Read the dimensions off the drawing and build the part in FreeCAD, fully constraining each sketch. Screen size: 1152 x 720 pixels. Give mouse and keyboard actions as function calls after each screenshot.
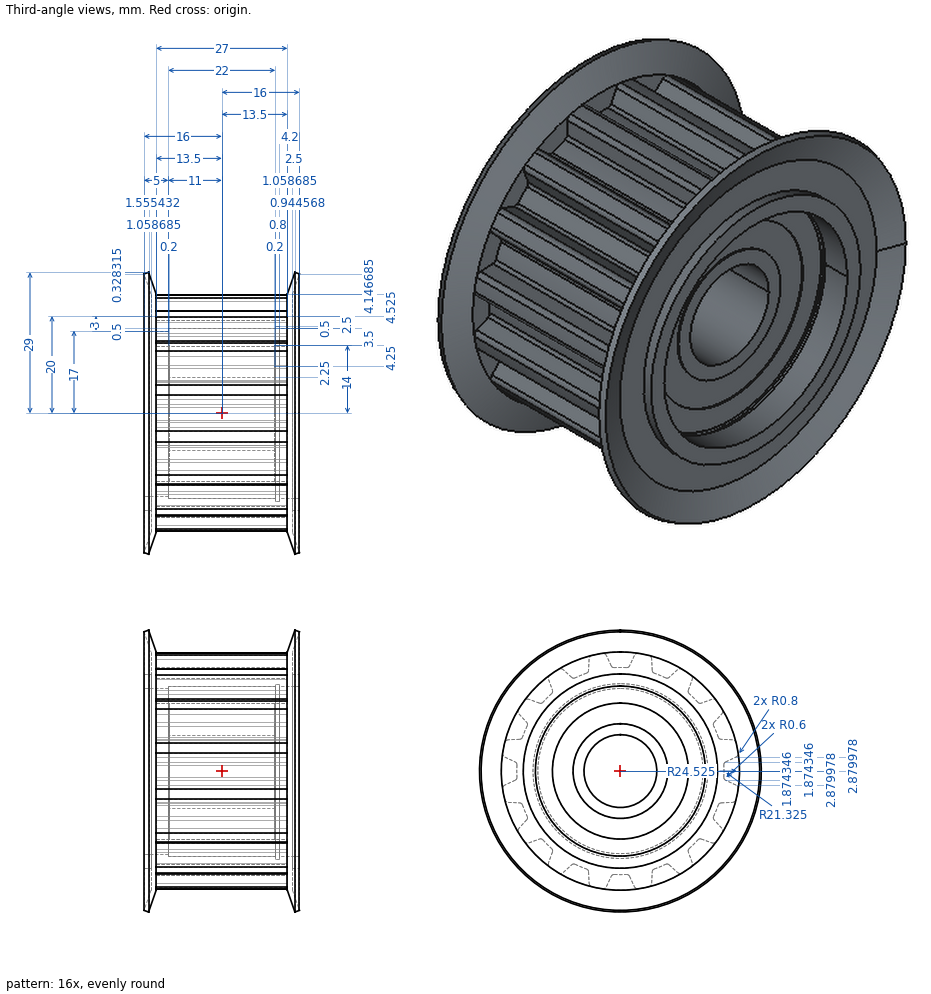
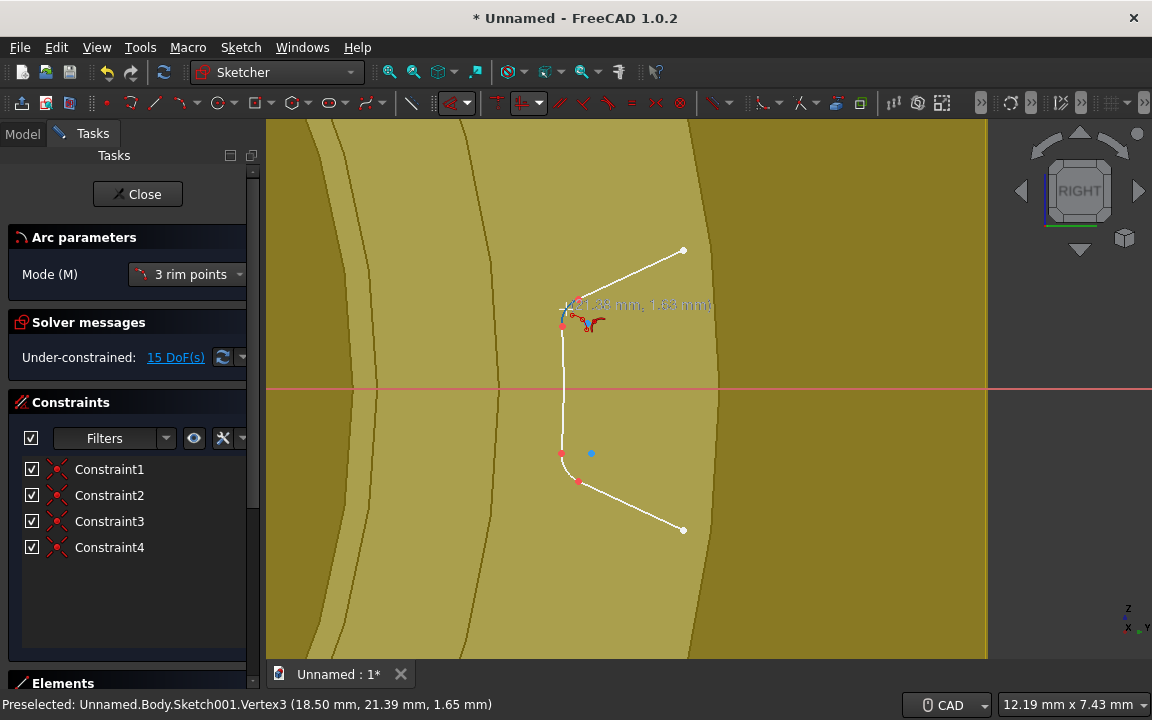
click(683, 250)
click(706, 208)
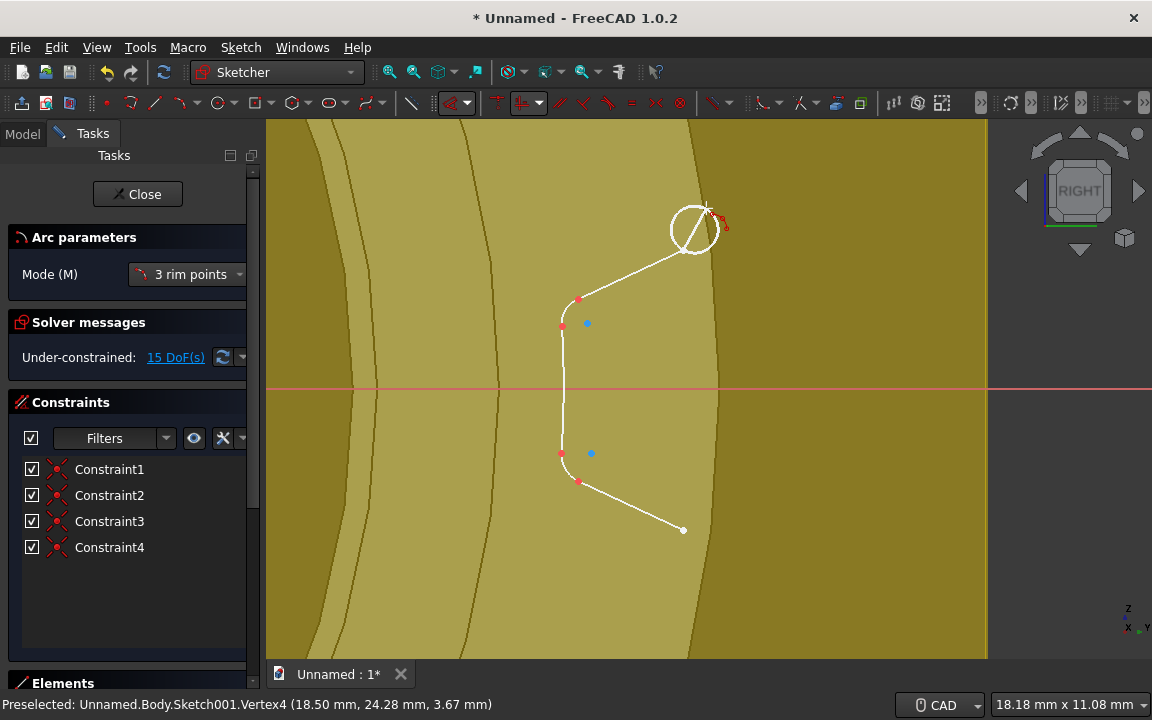
scroll(702, 232, up, 4)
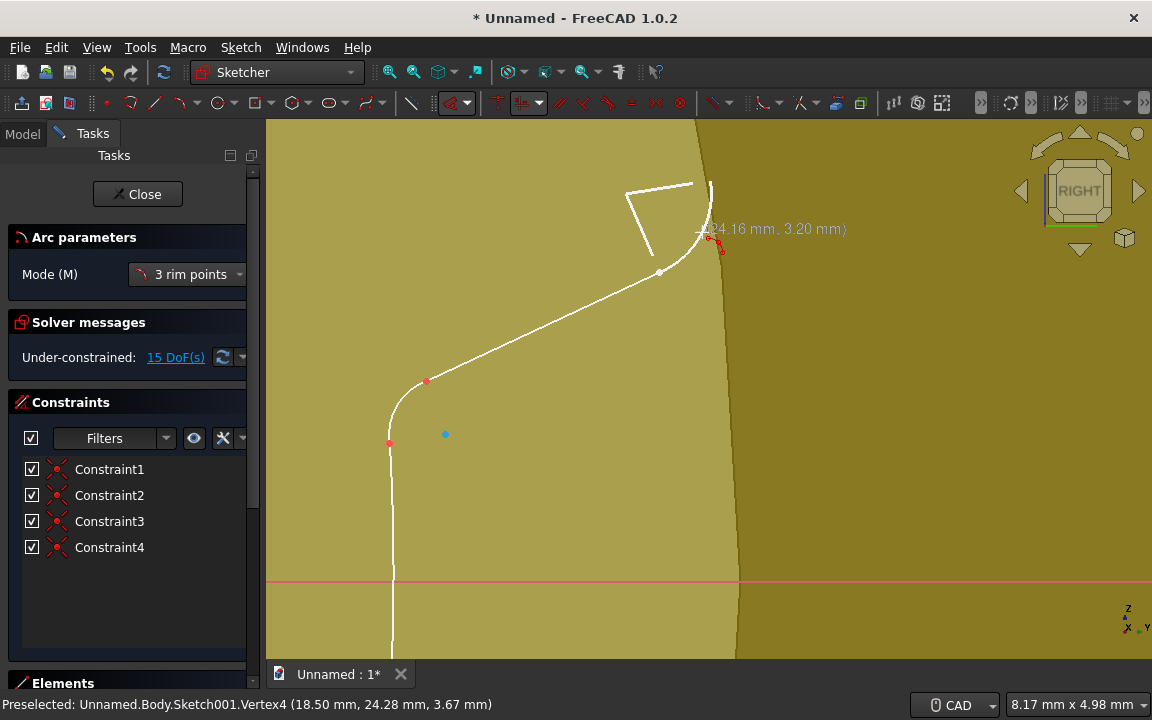
click(700, 231)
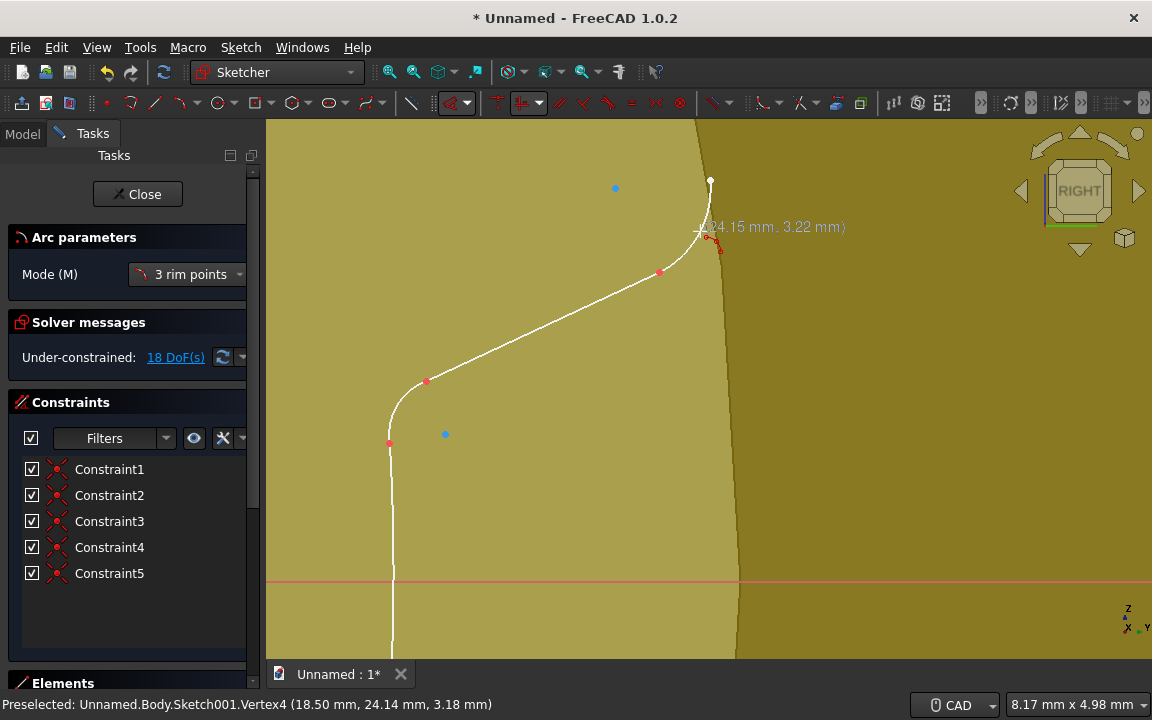
click(710, 181)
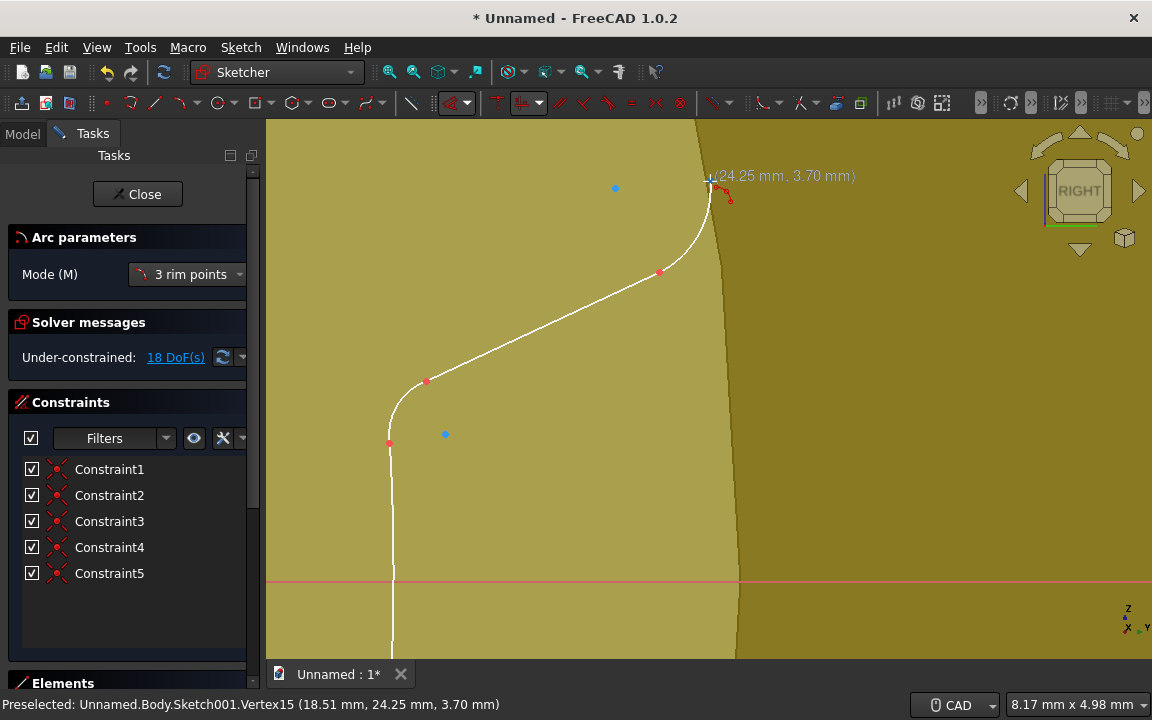
scroll(702, 232, down, 4)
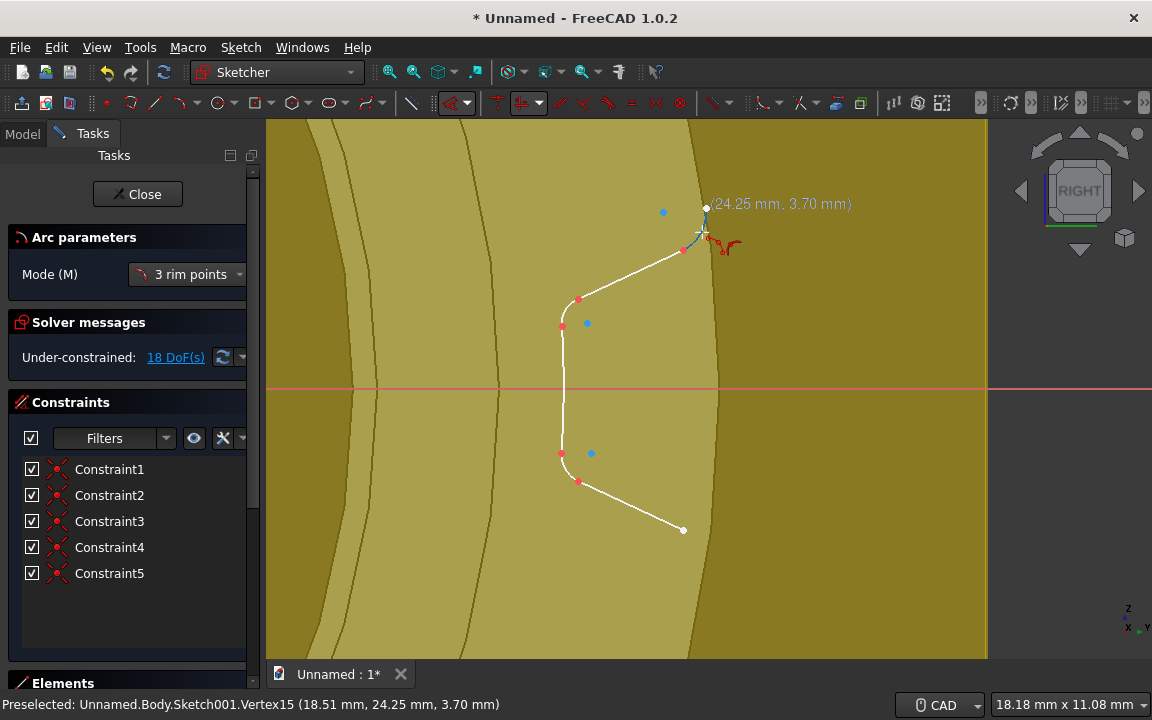
click(706, 571)
click(719, 426)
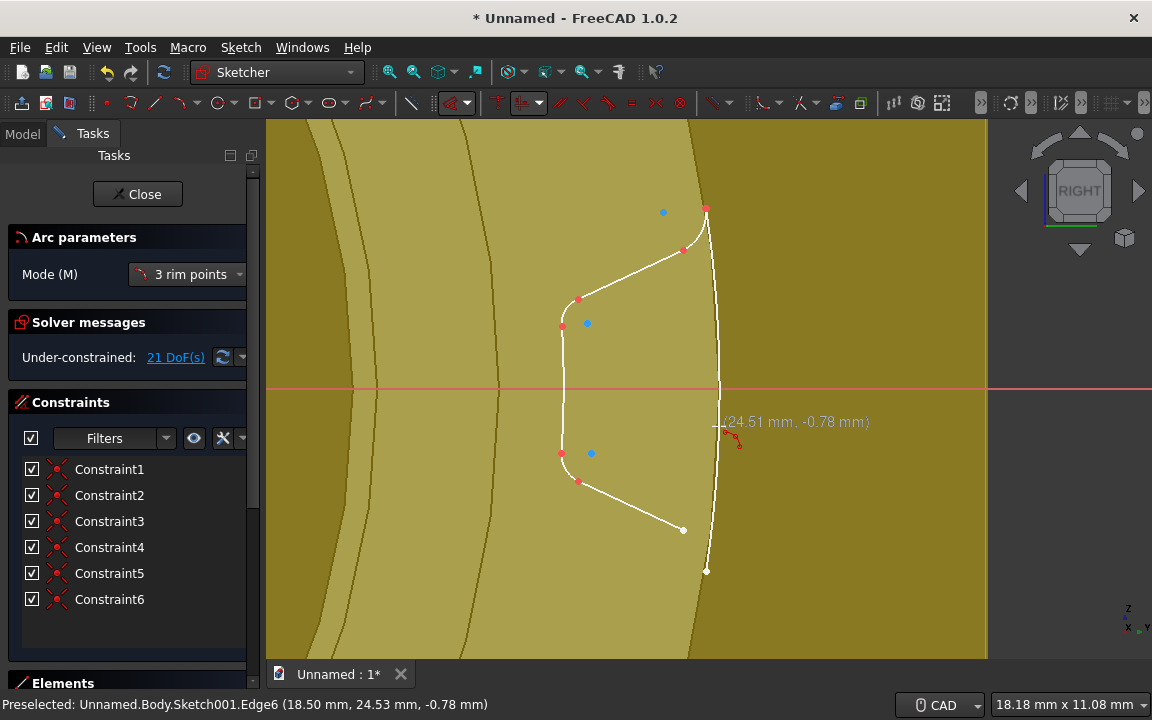
click(706, 572)
click(683, 530)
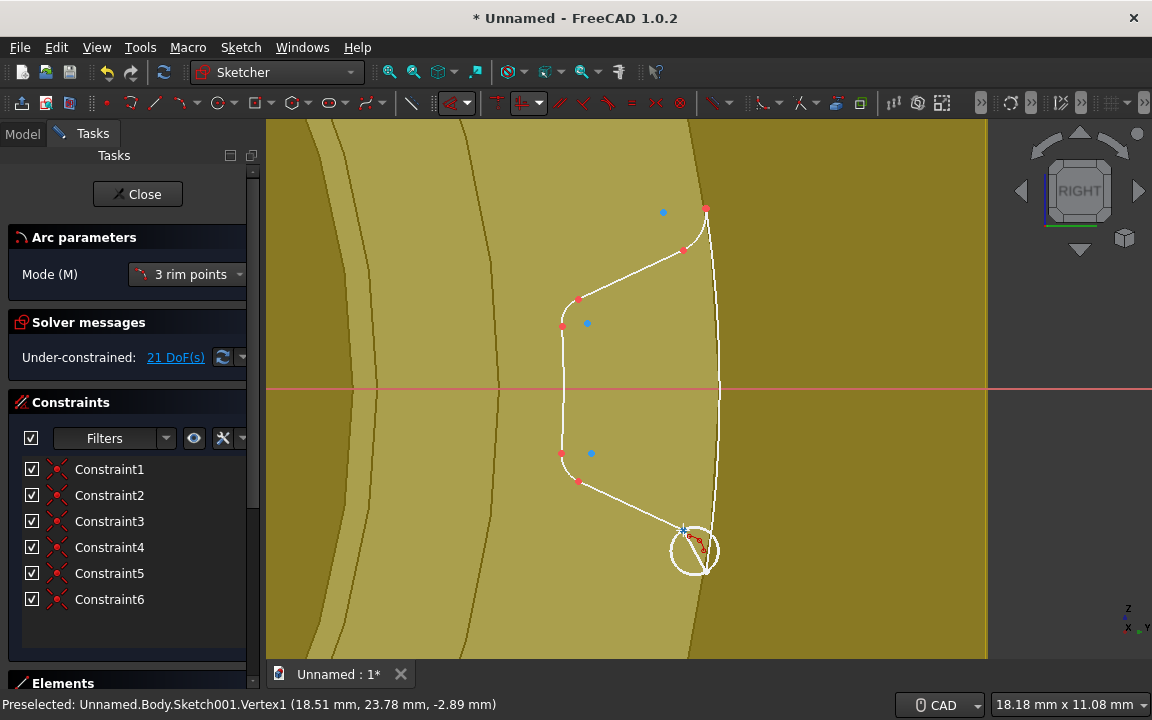
scroll(702, 546, up, 4)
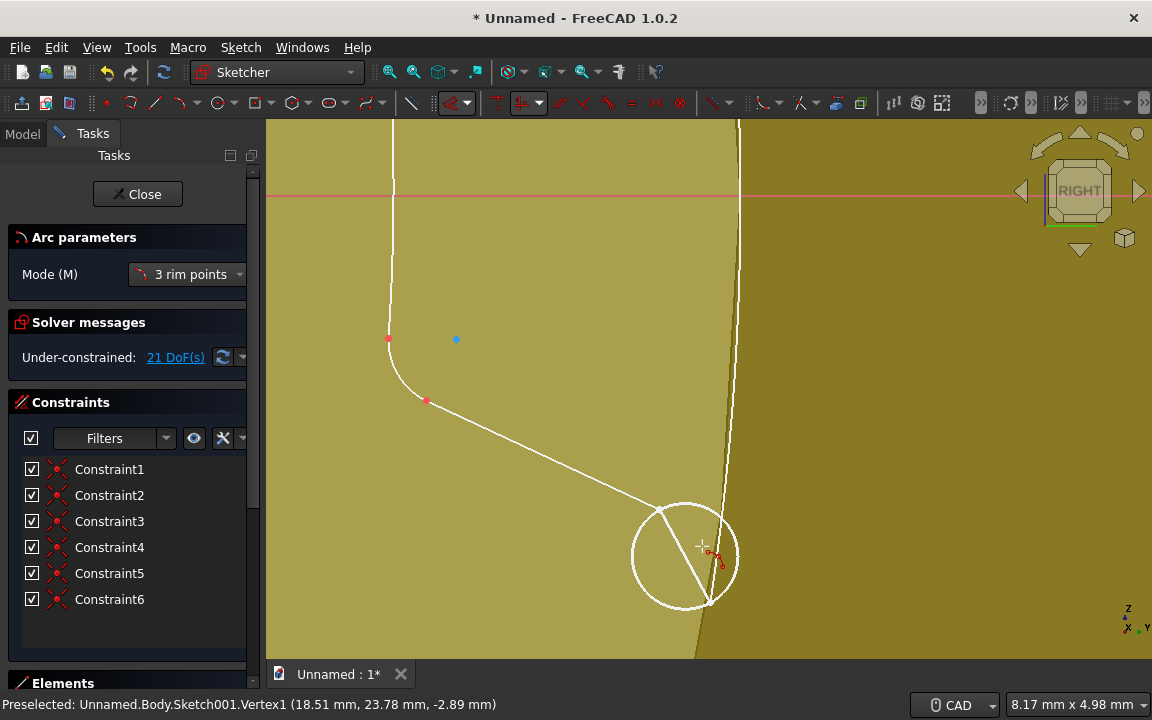
click(700, 546)
key(Escape)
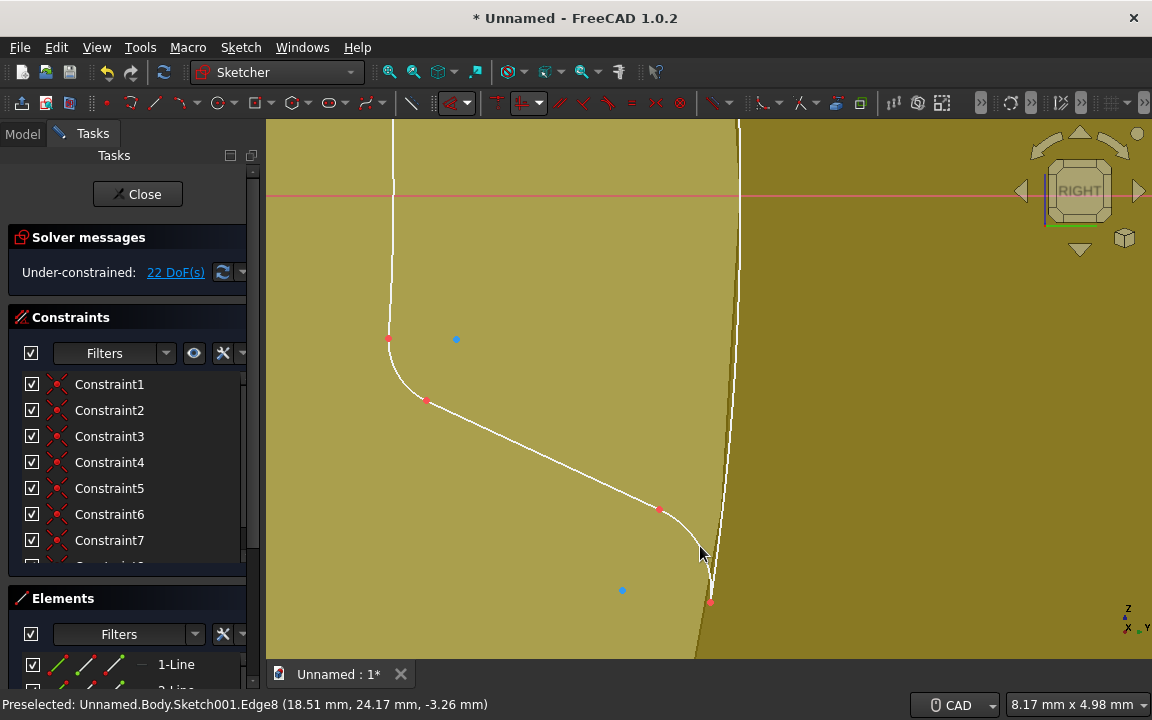
click(590, 477)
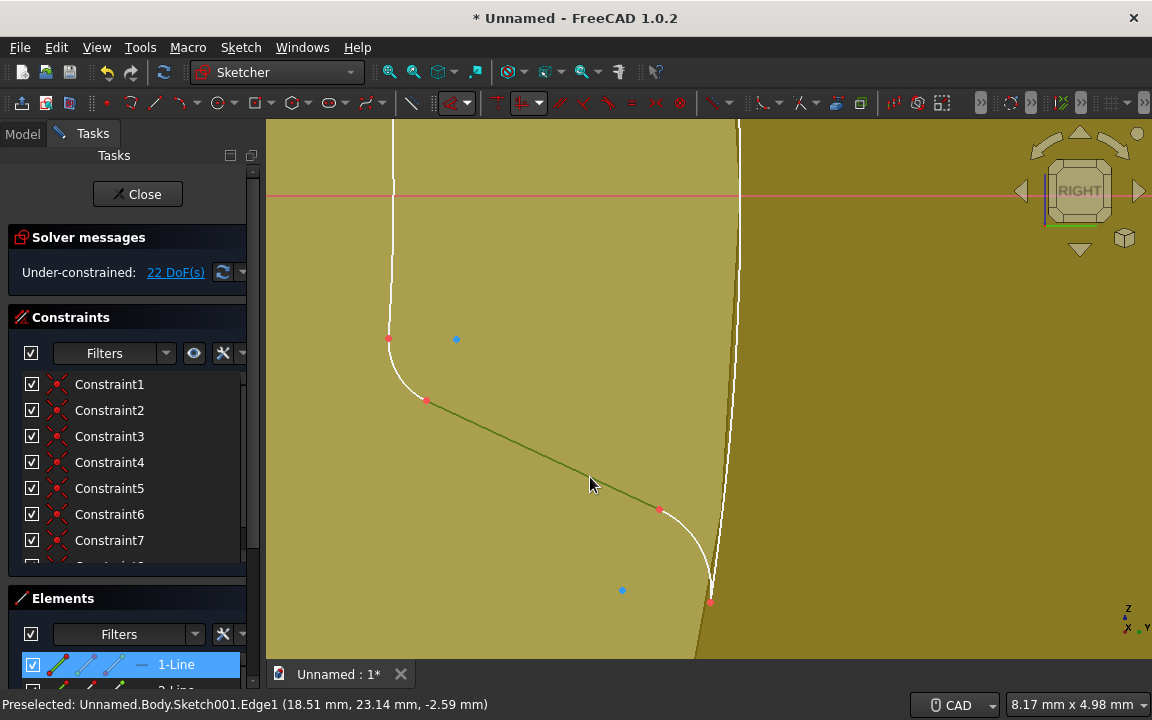
click(392, 361)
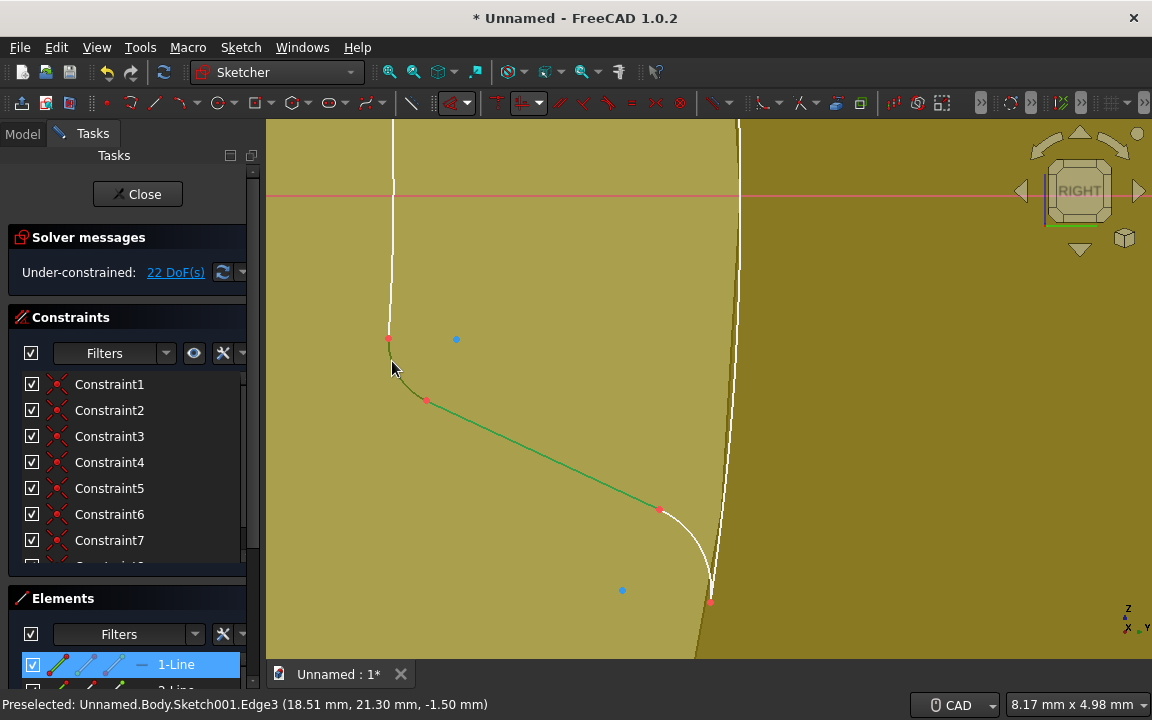
click(608, 104)